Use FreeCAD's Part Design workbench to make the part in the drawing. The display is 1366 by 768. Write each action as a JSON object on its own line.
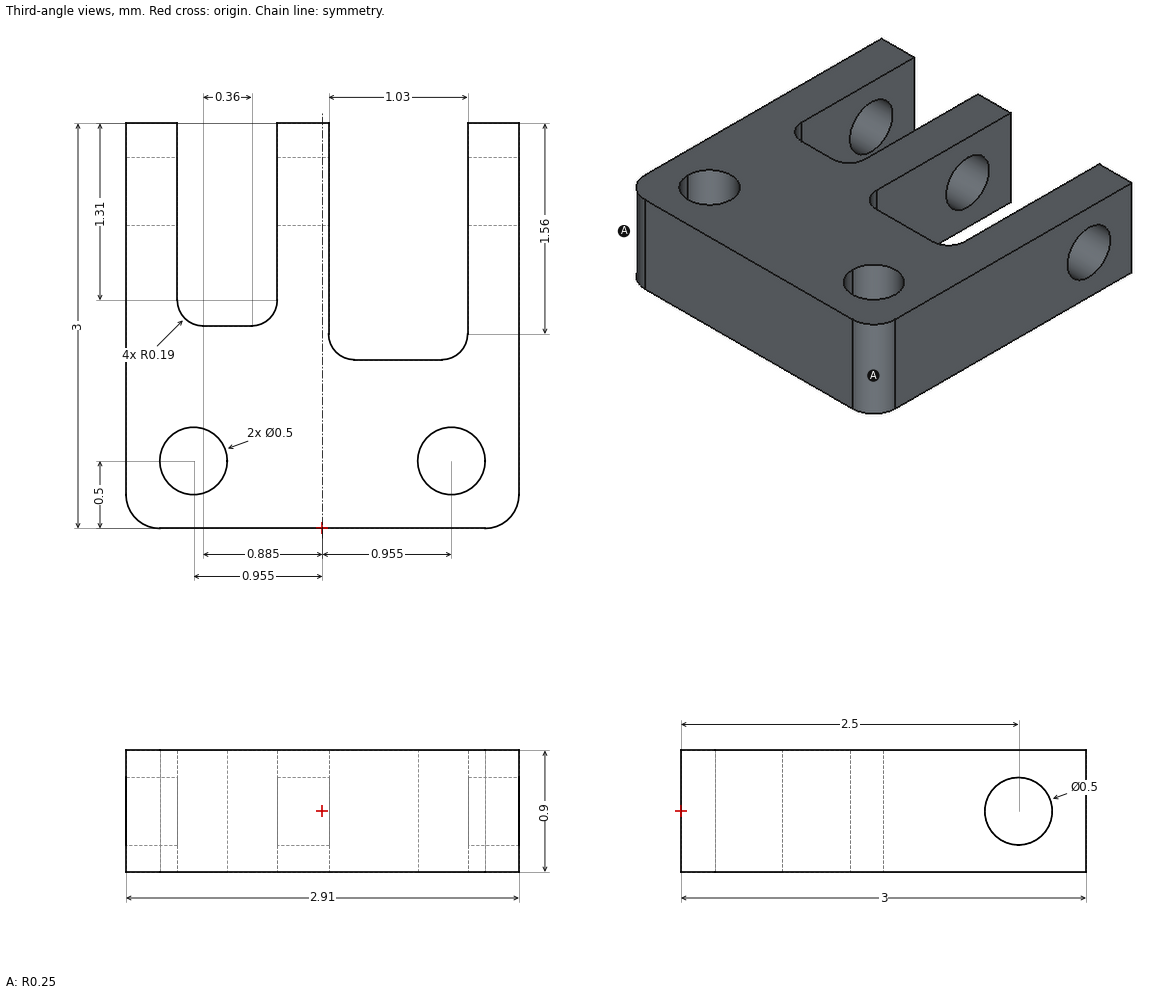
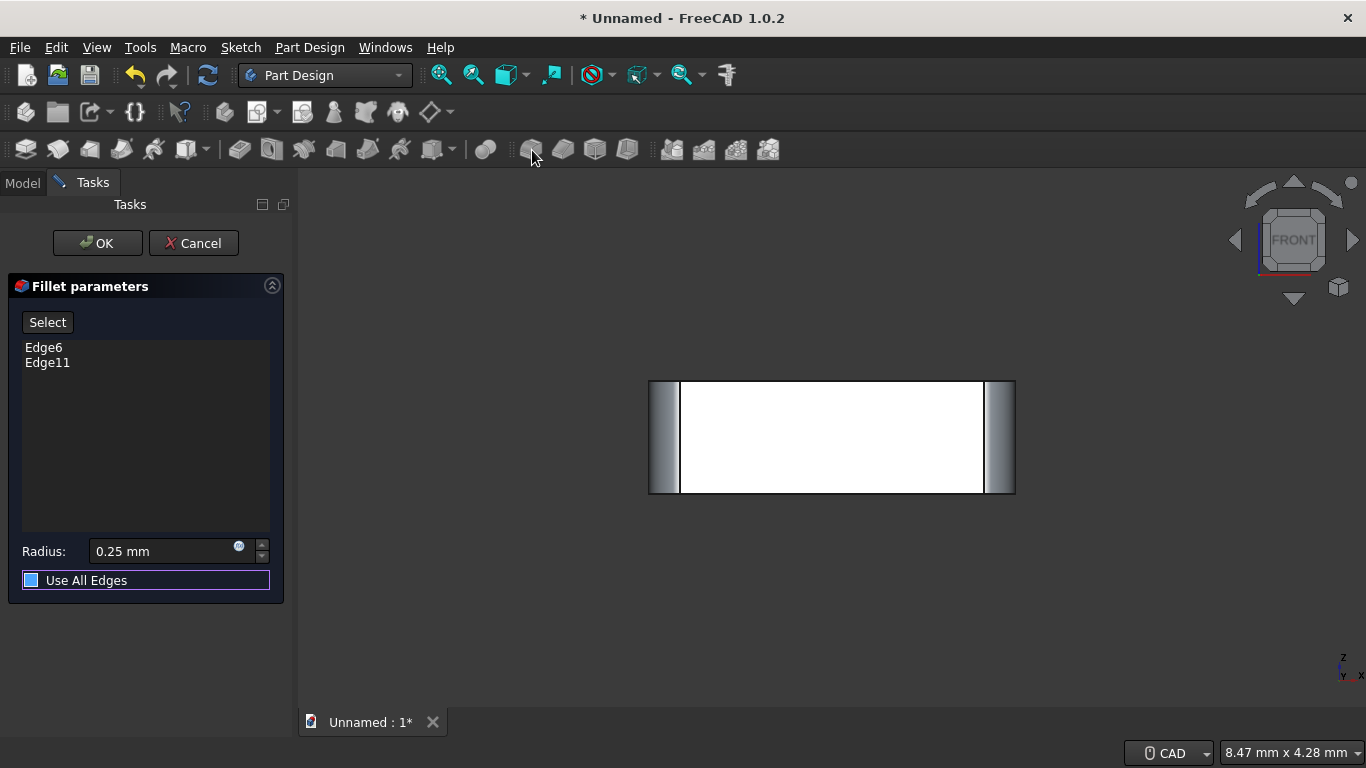
{"action": "left_click", "coordinate": [98, 243]}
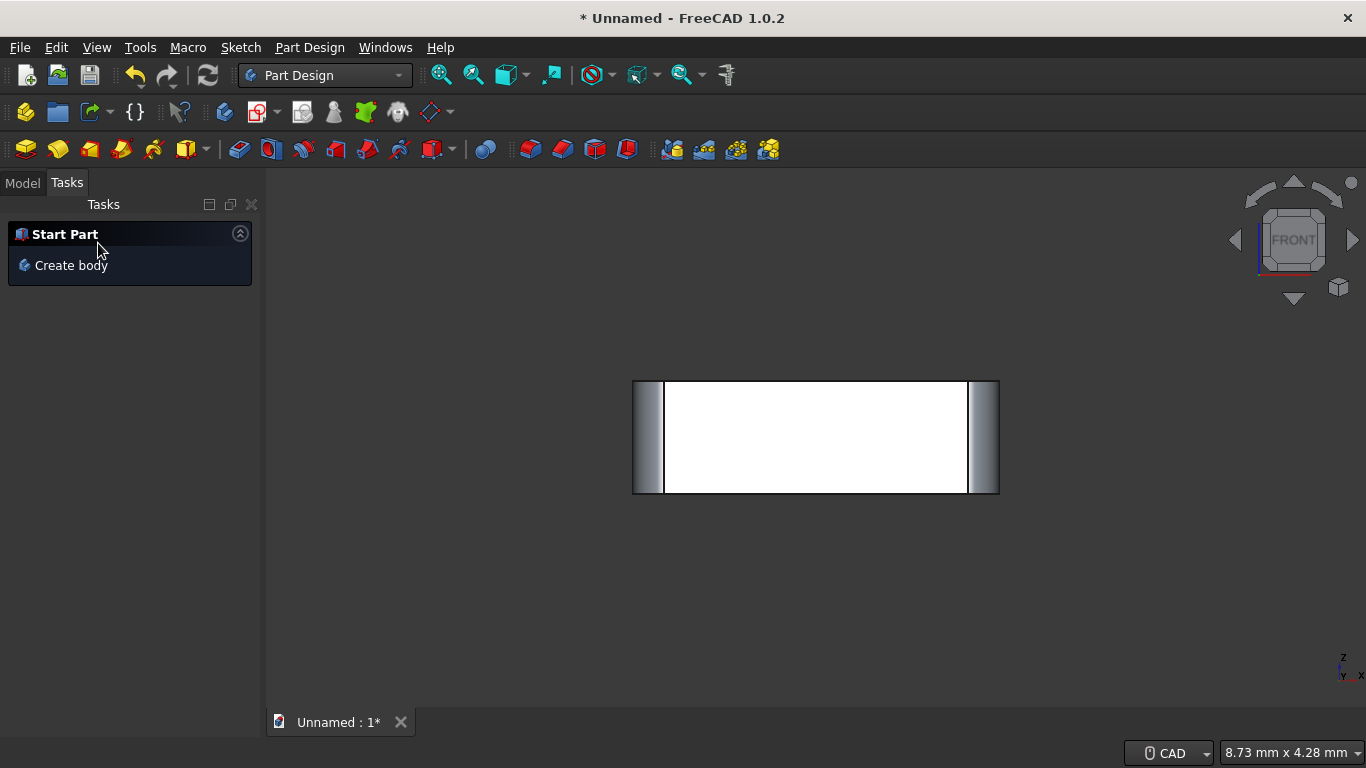
{"action": "key", "text": "v f"}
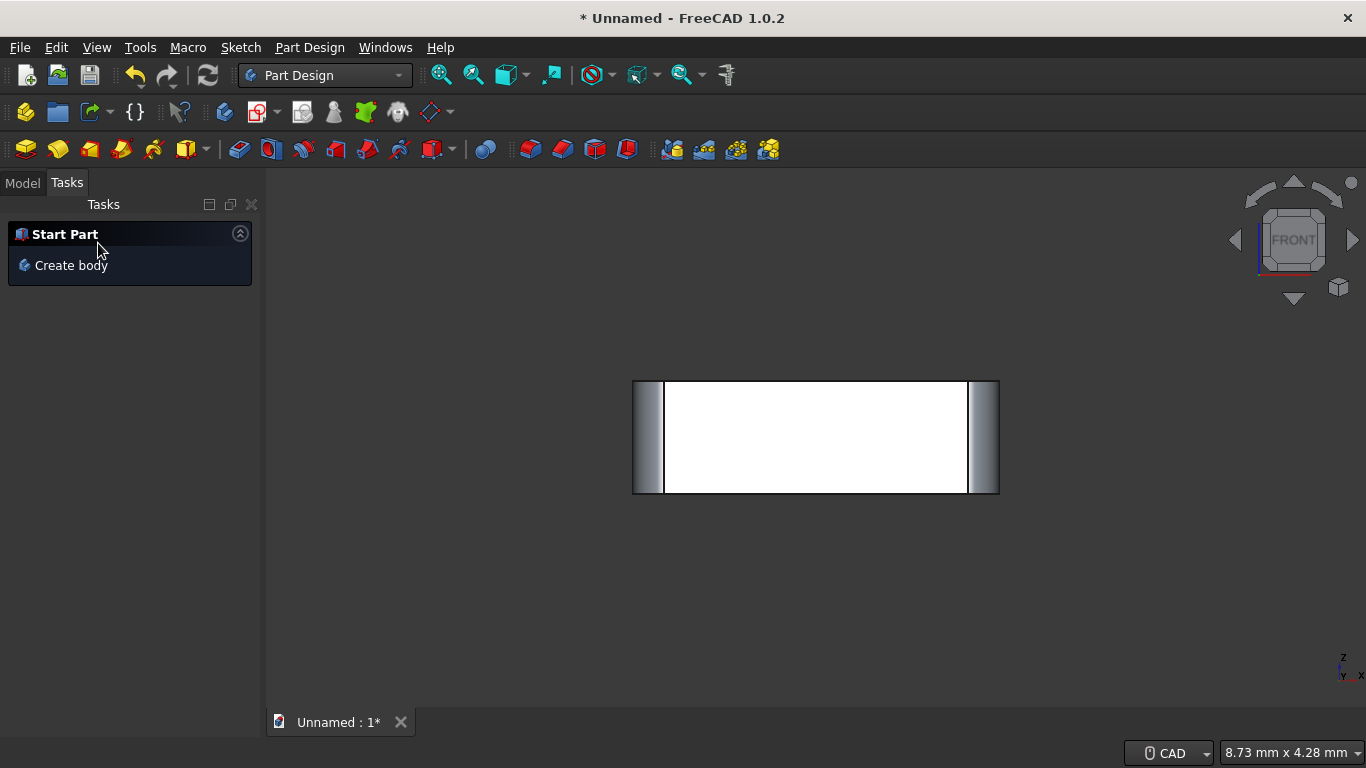
{"action": "key", "text": "0"}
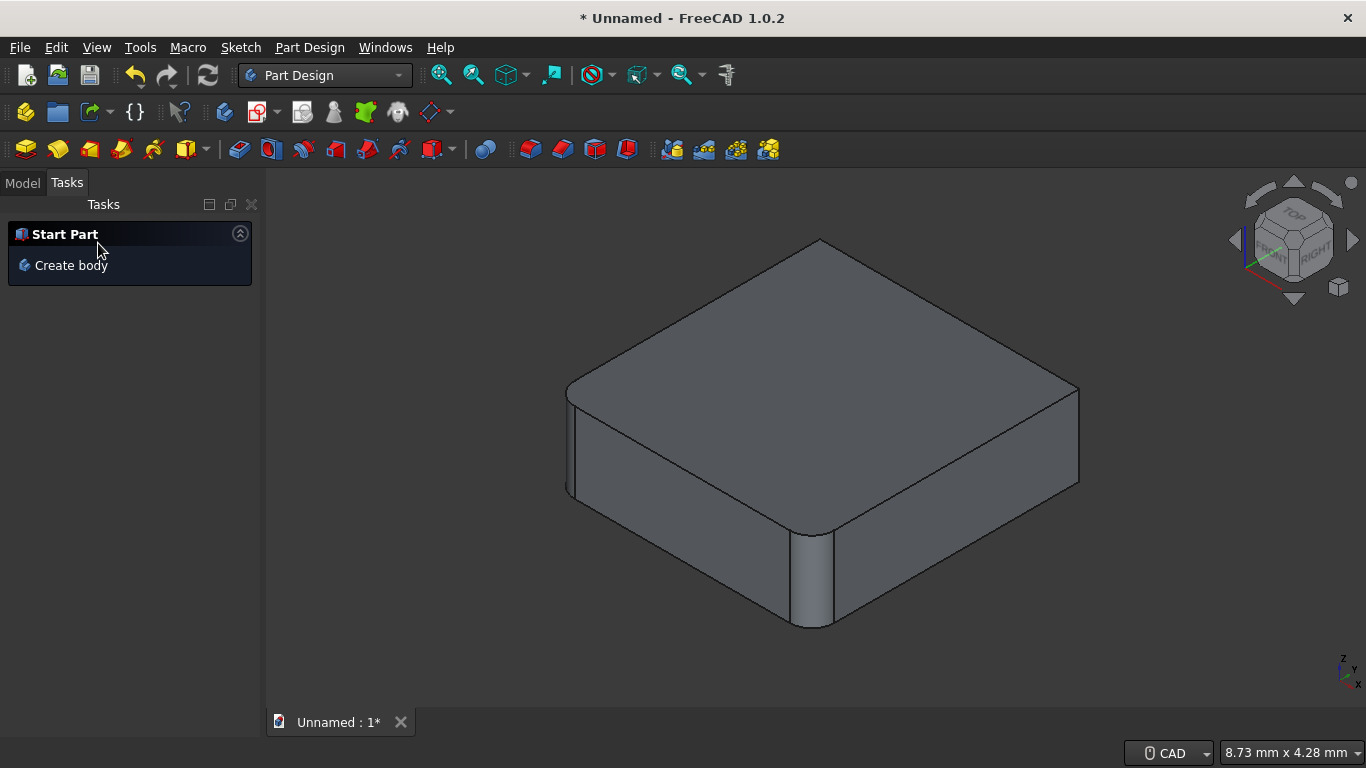
{"action": "left_click", "coordinate": [816, 390]}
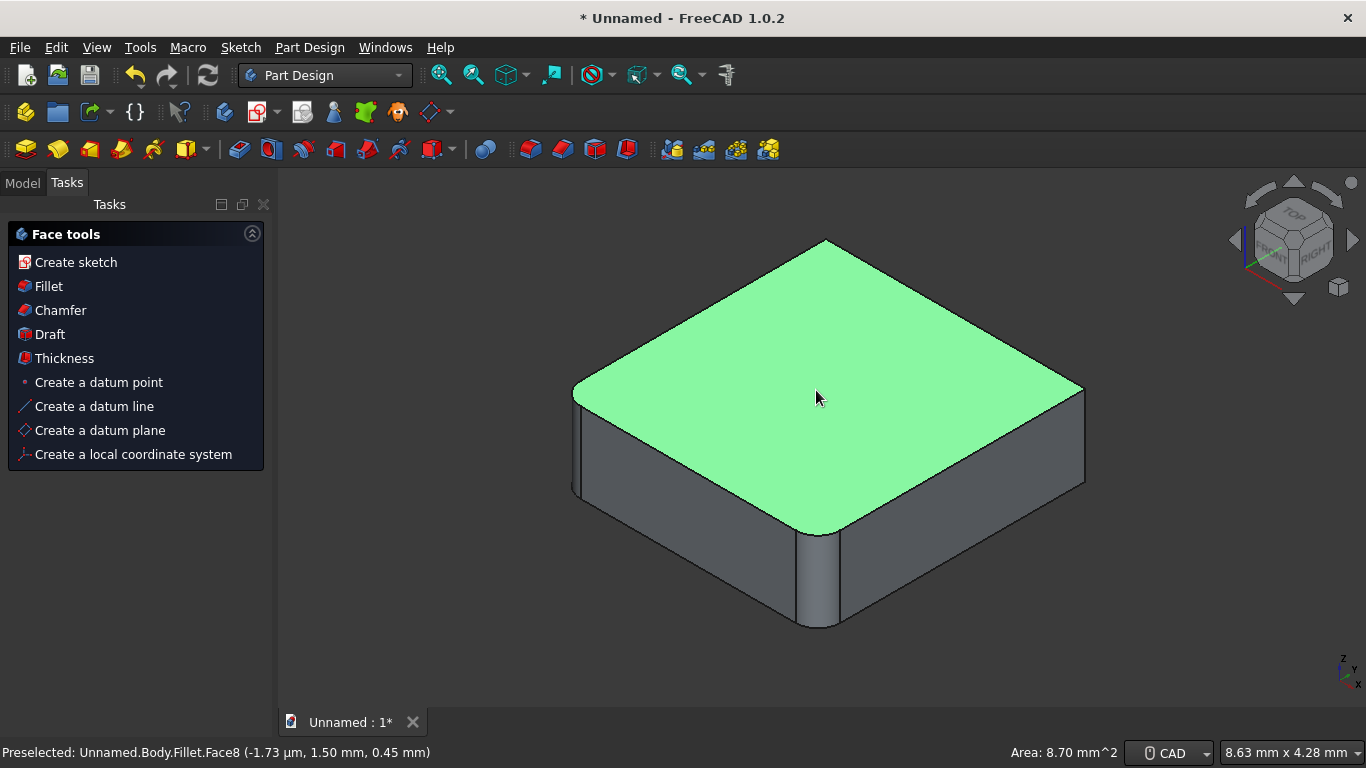
{"action": "left_click", "coordinate": [258, 112]}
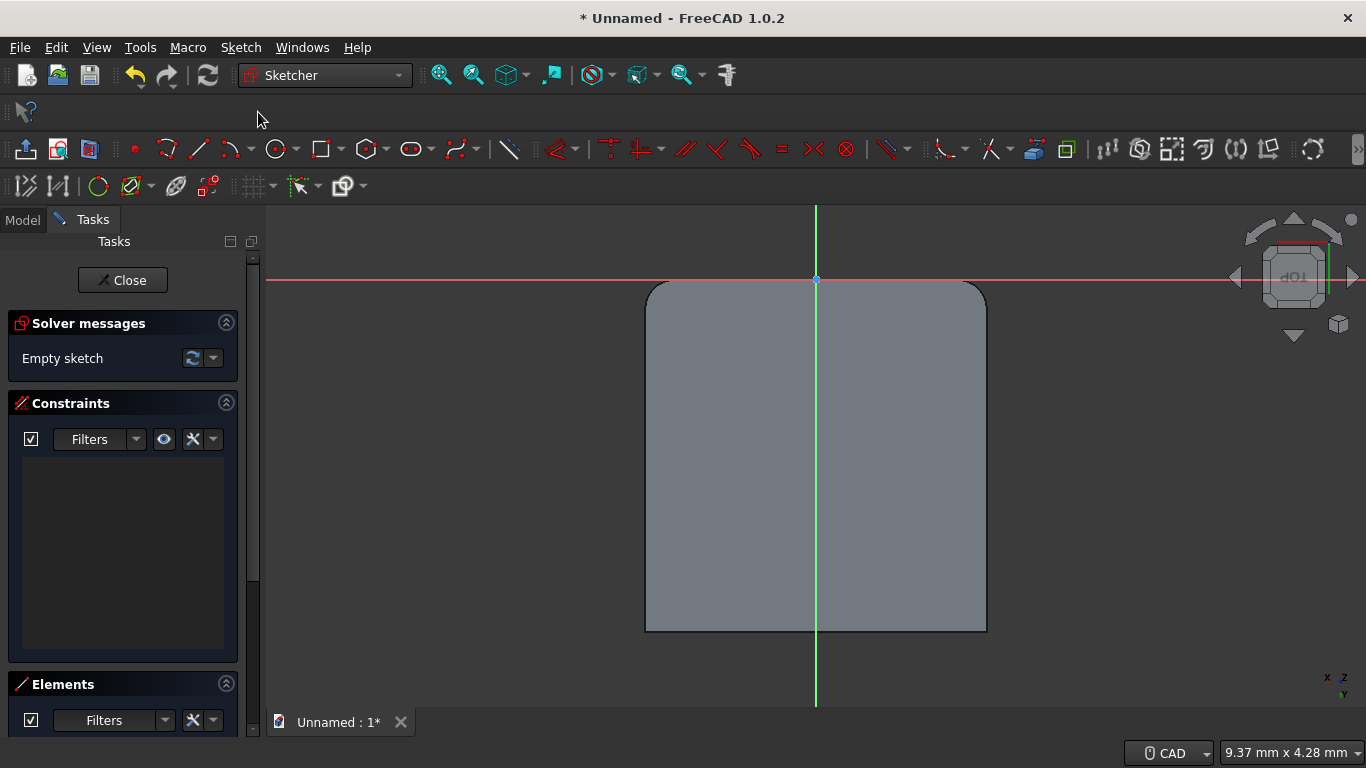
{"action": "key", "text": "g l"}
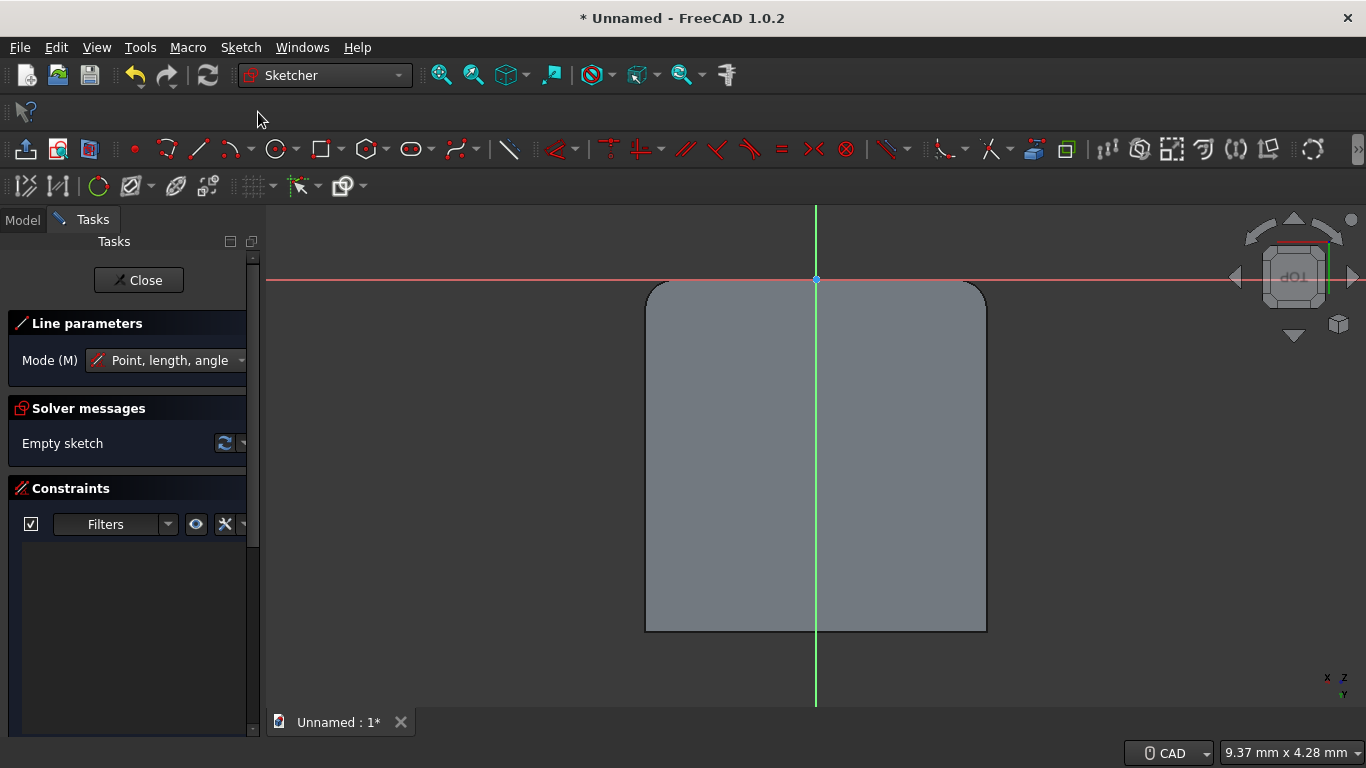
{"action": "left_click", "coordinate": [920, 456]}
{"action": "left_click", "coordinate": [878, 456]}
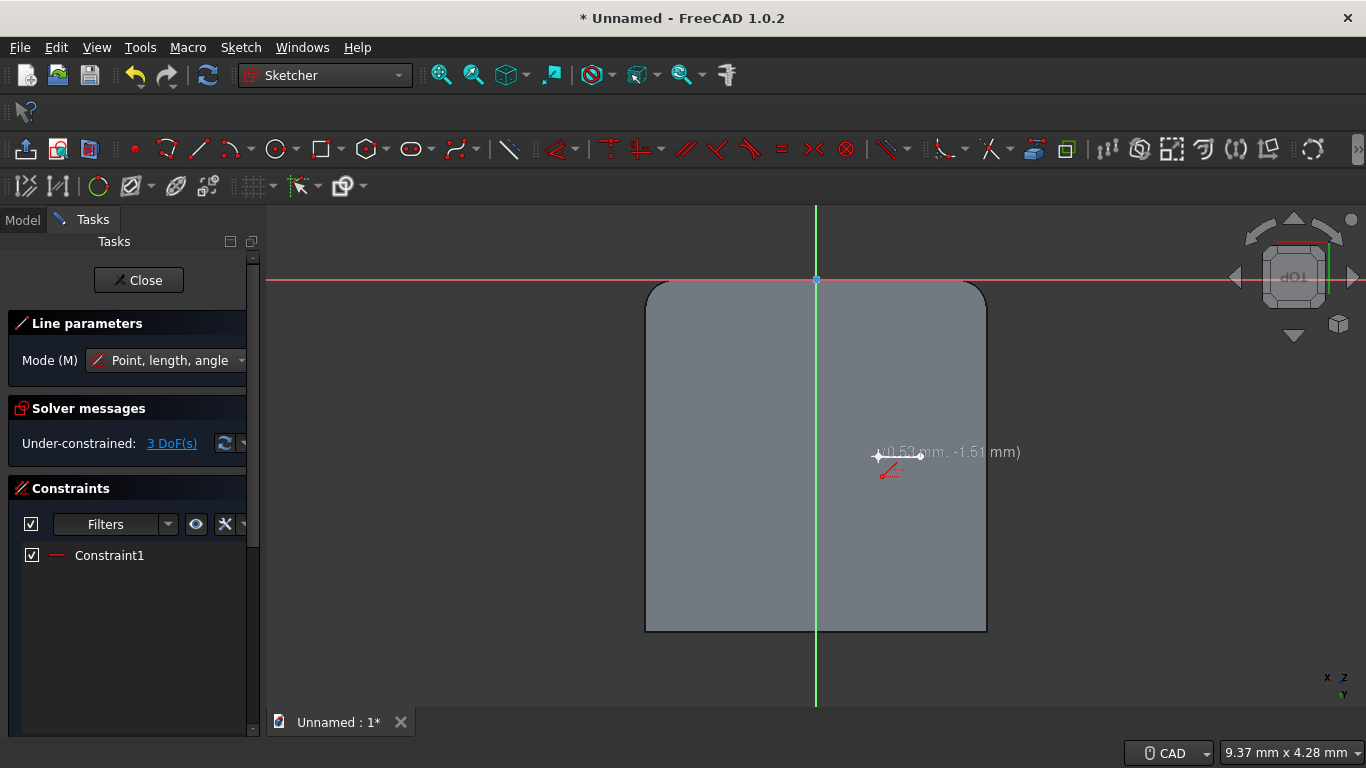
{"action": "left_click", "coordinate": [168, 150]}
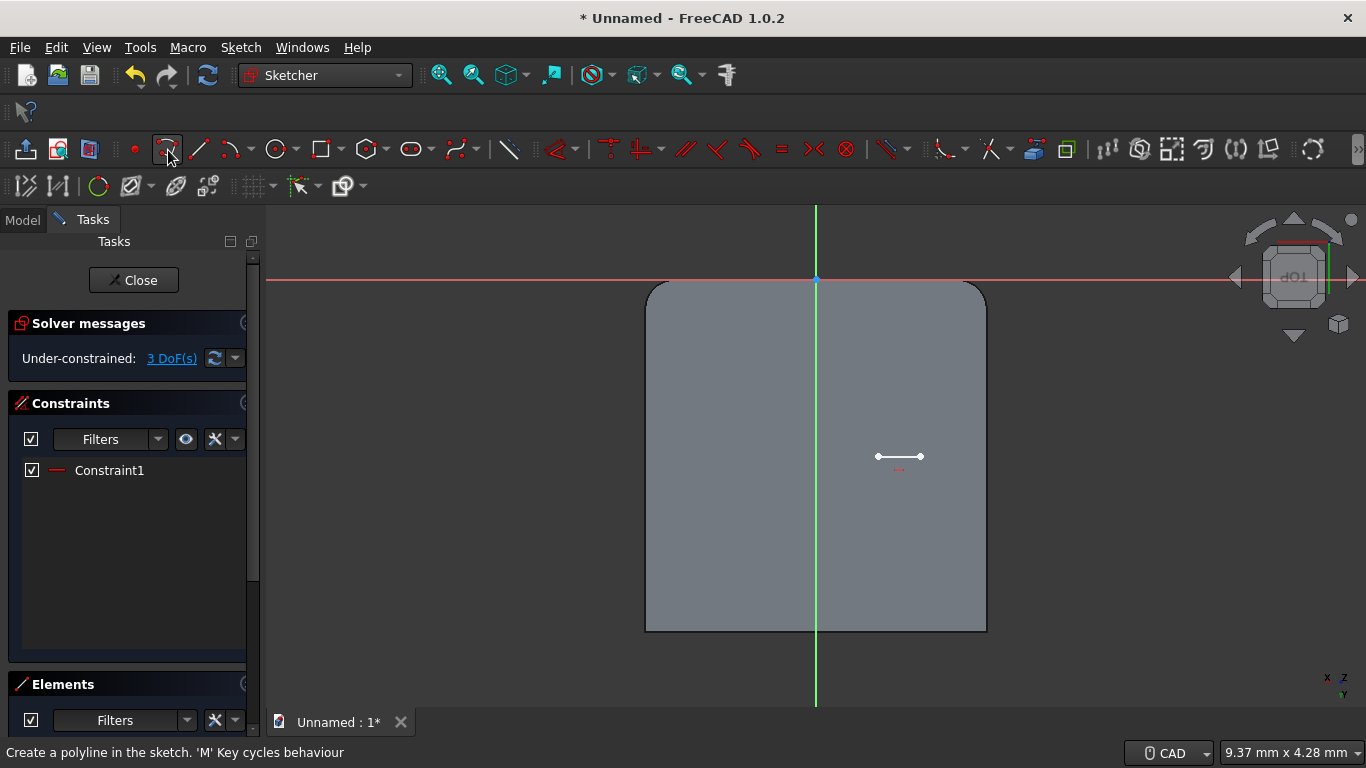
{"action": "left_click", "coordinate": [855, 478]}
{"action": "left_click", "coordinate": [855, 632]}
{"action": "left_click", "coordinate": [942, 632]}
{"action": "left_click", "coordinate": [942, 478]}
{"action": "right_click", "coordinate": [942, 478]}